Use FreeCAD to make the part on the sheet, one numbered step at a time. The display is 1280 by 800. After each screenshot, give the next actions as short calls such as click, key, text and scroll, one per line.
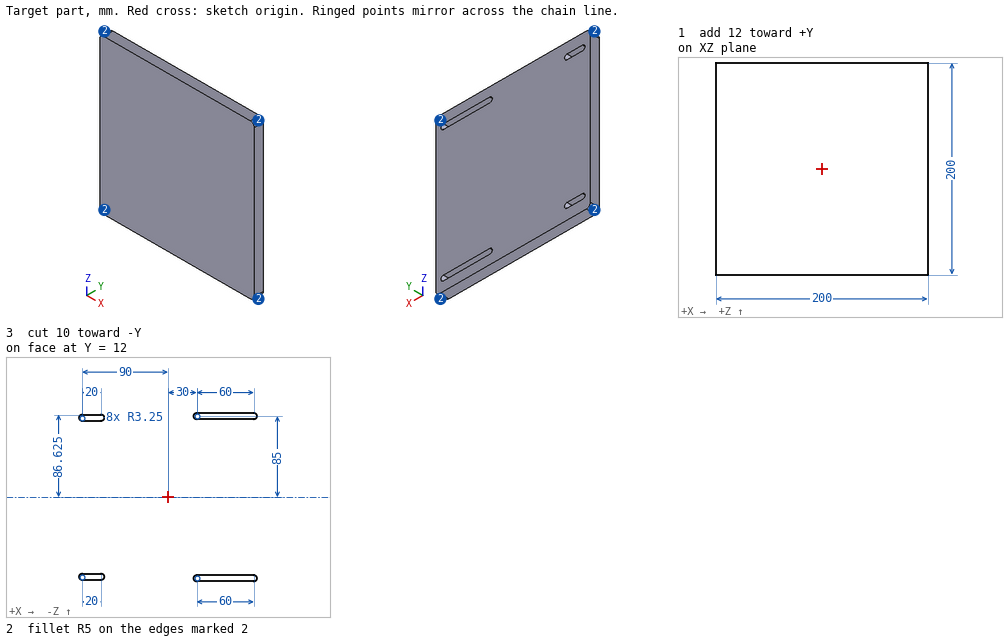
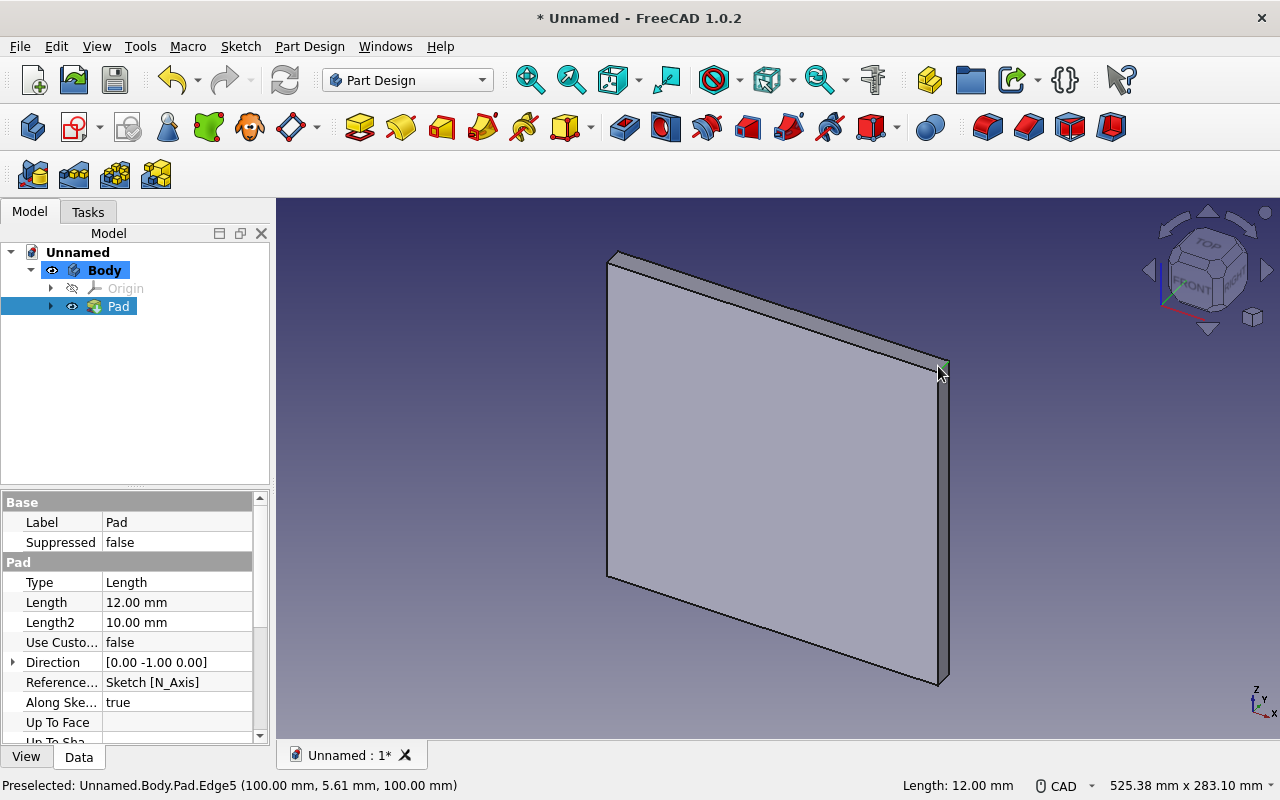
key(0)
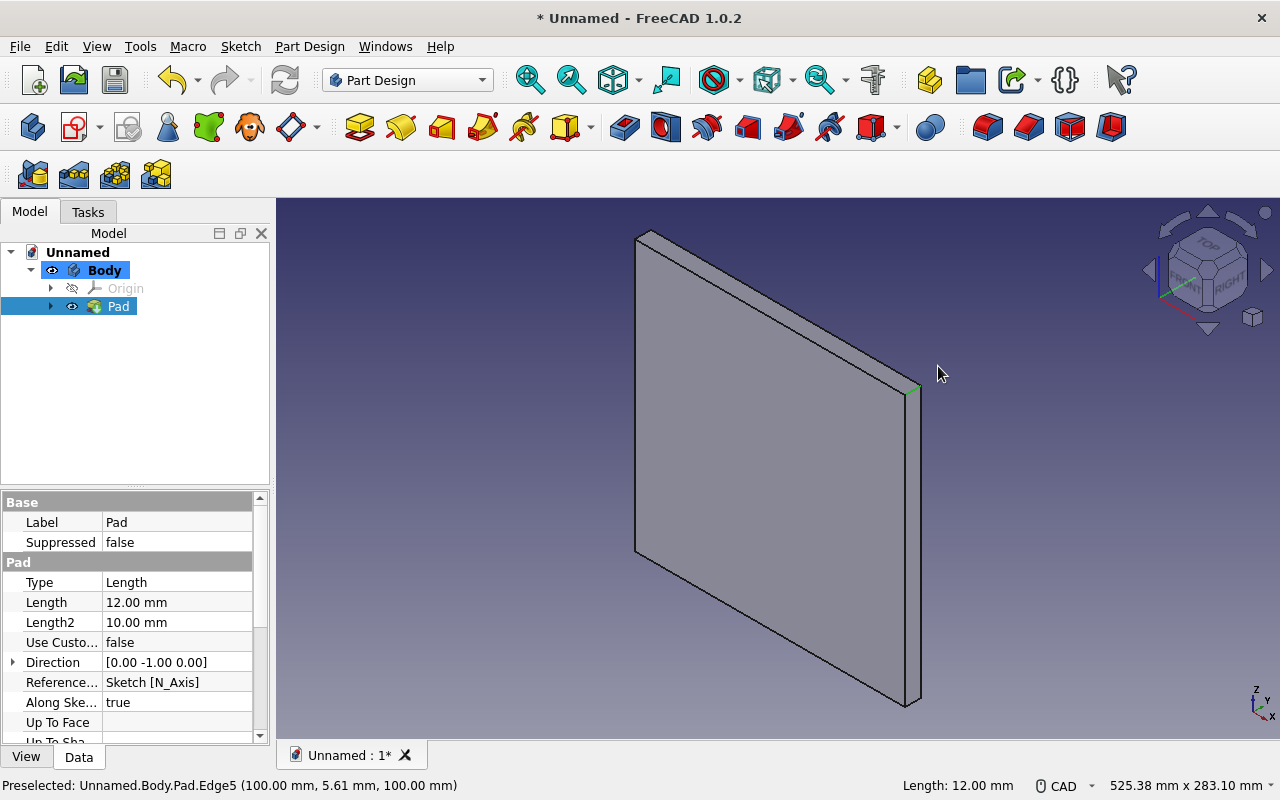
key(2)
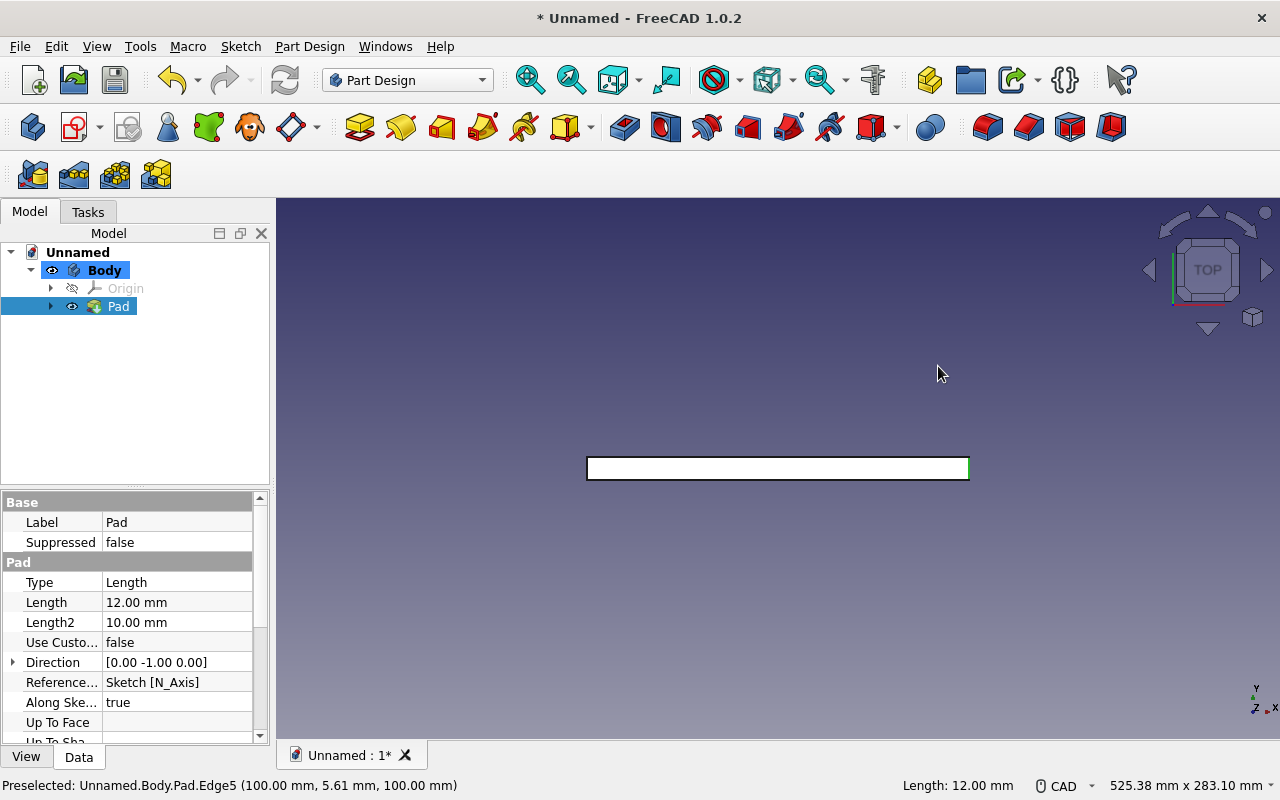
click(531, 80)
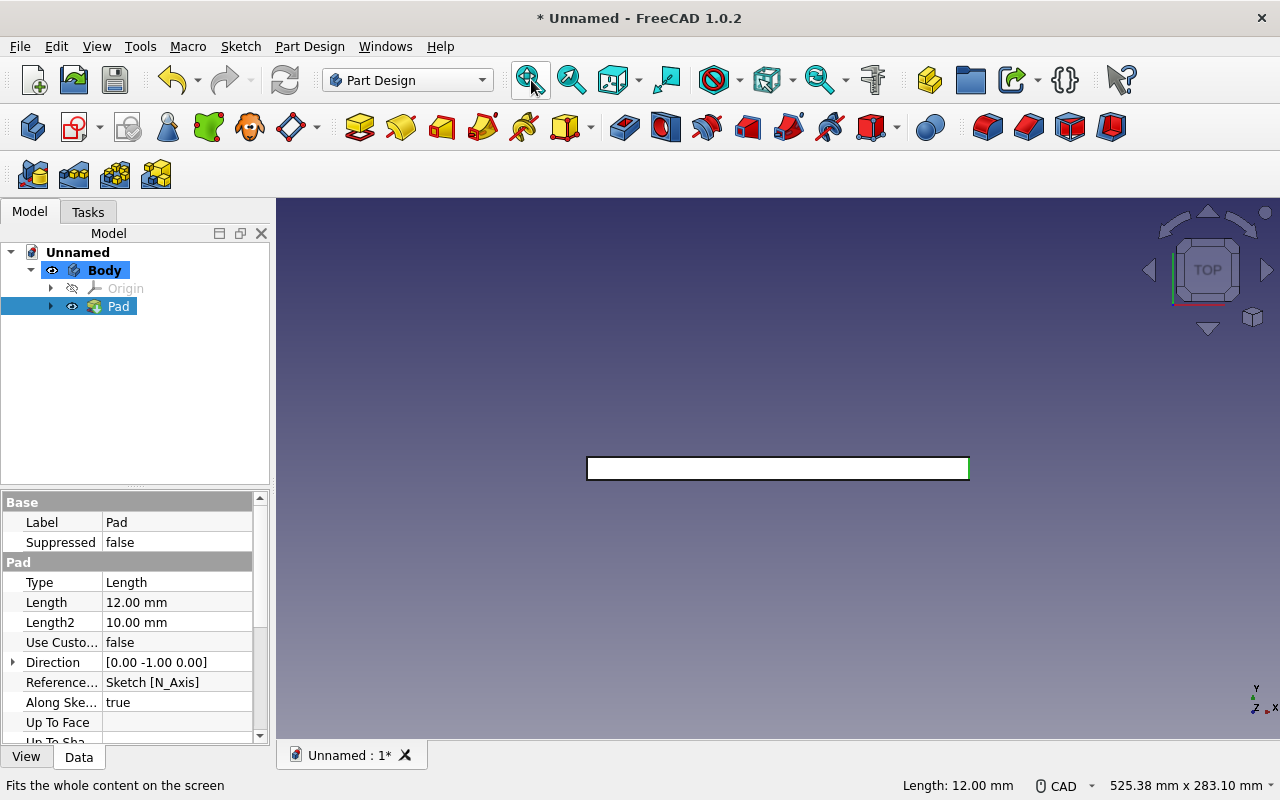
click(587, 467, ctrl)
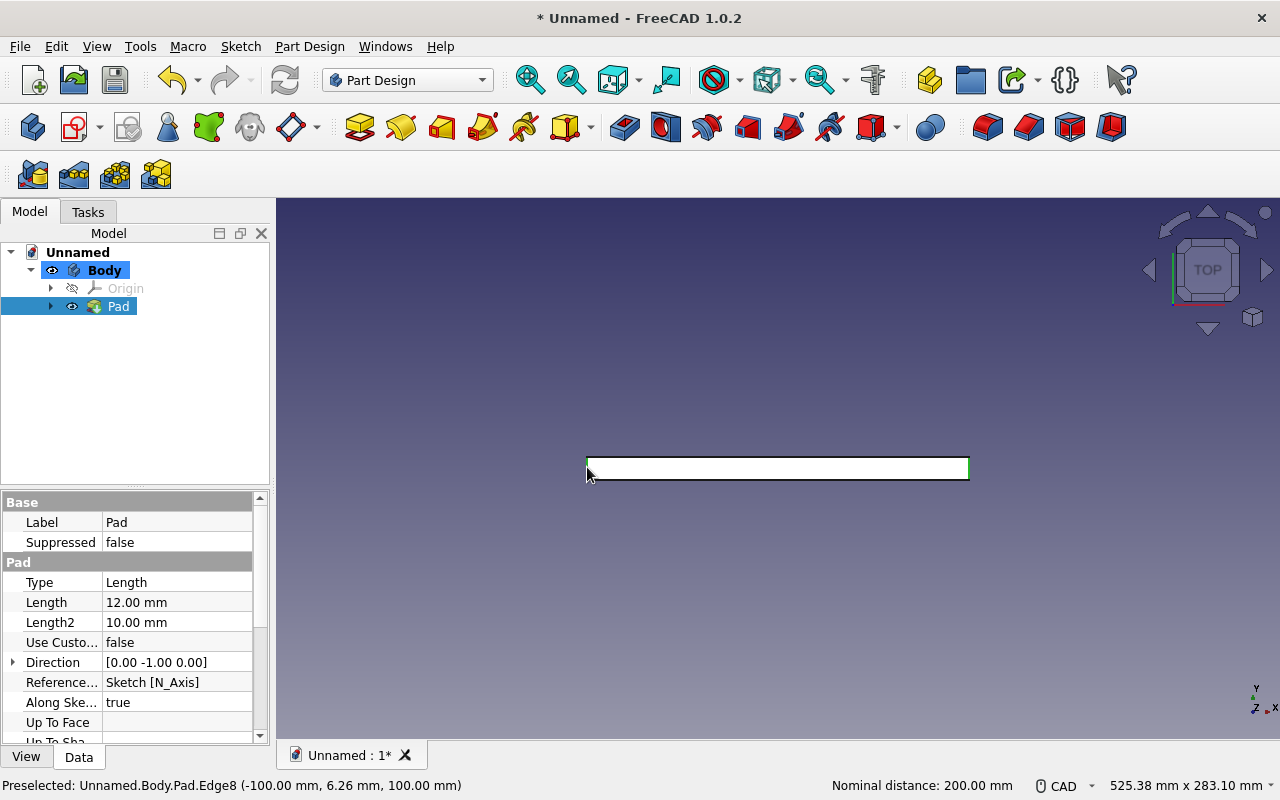
key(1)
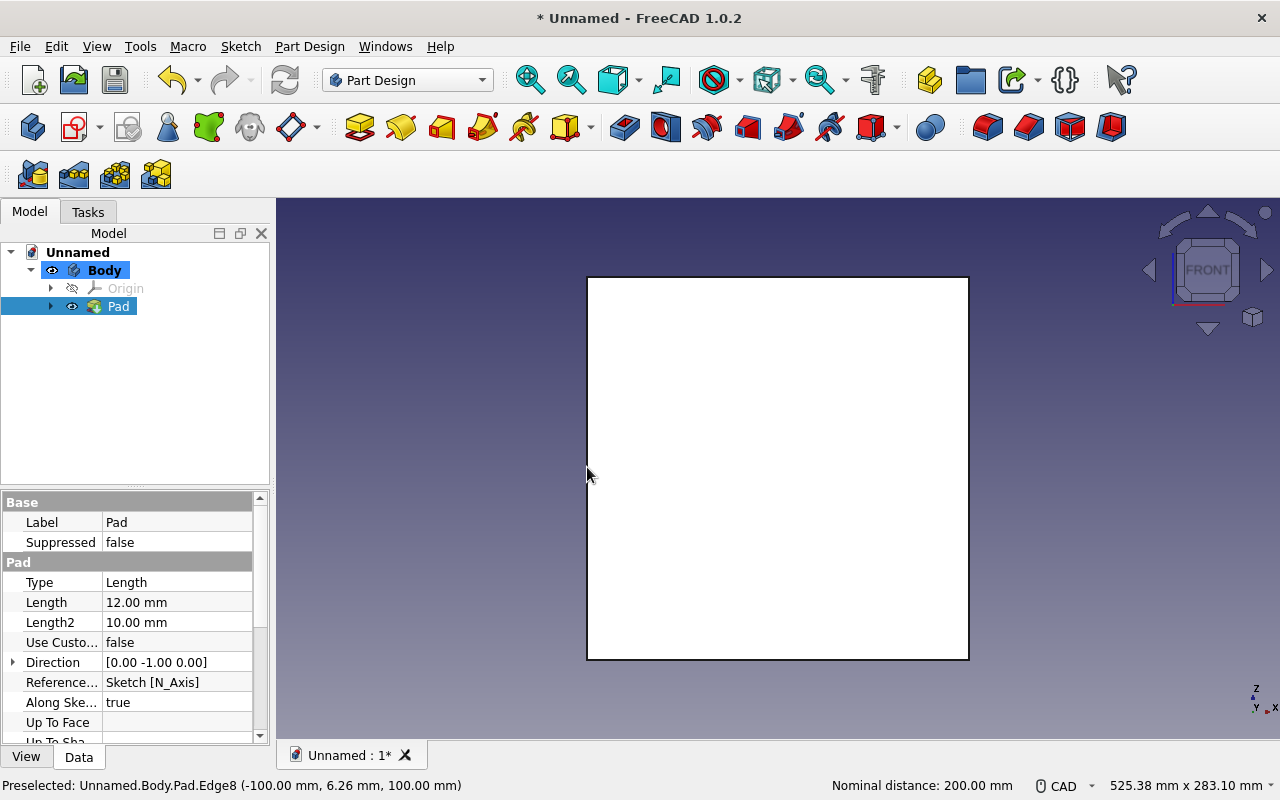
key(3)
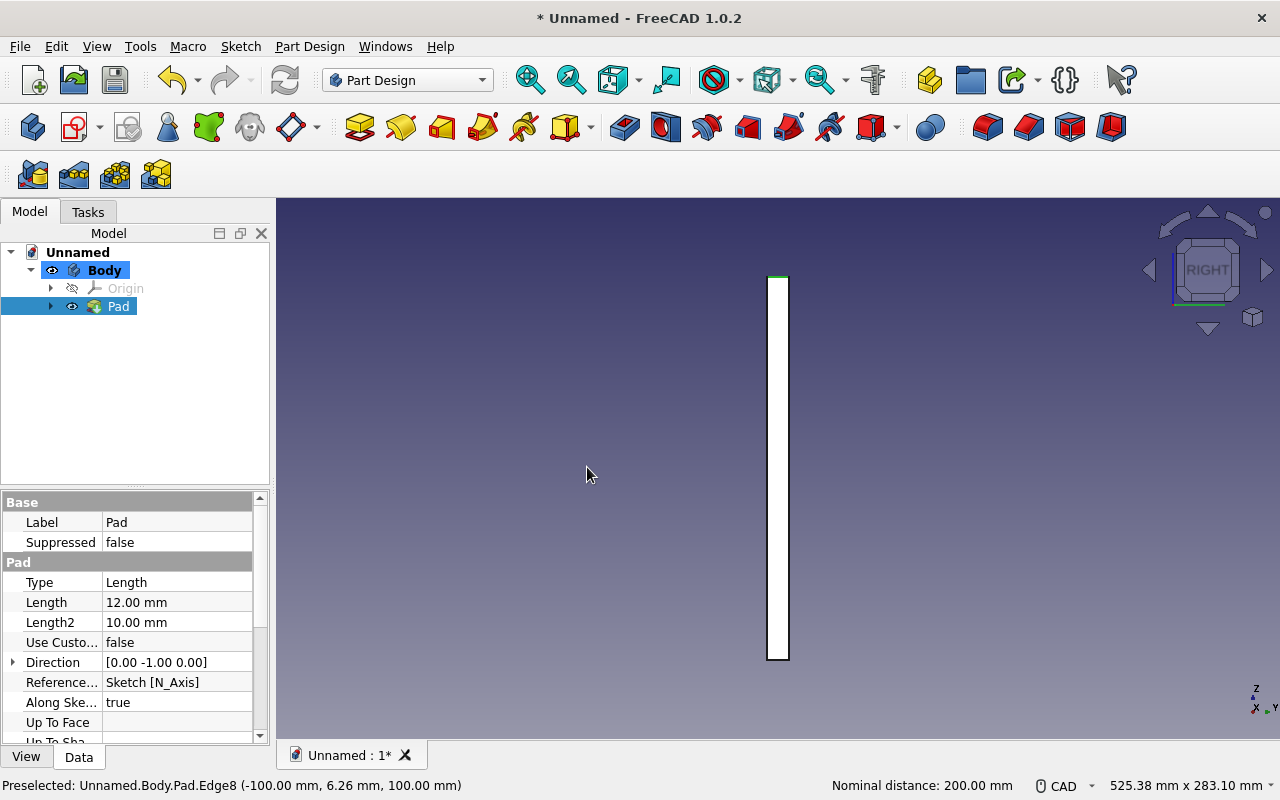
click(778, 659, ctrl)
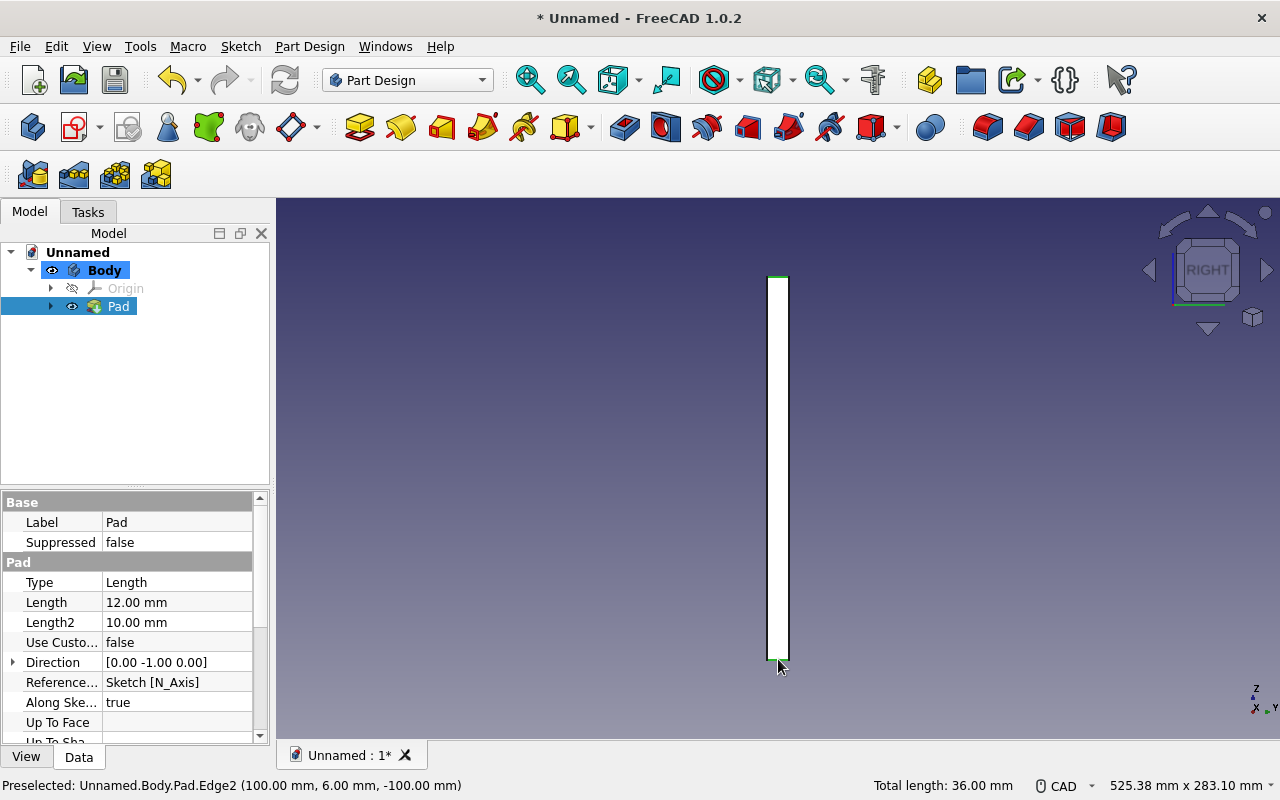
key(5)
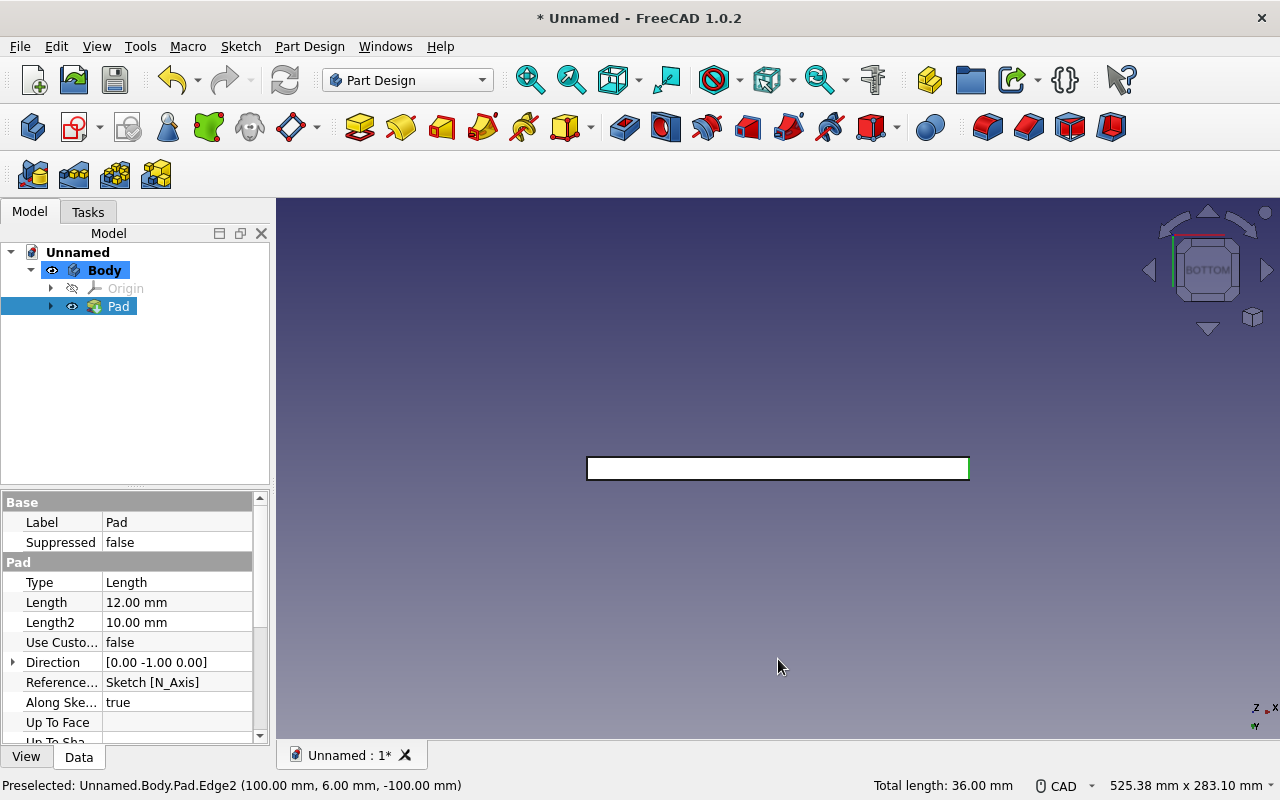
click(531, 80)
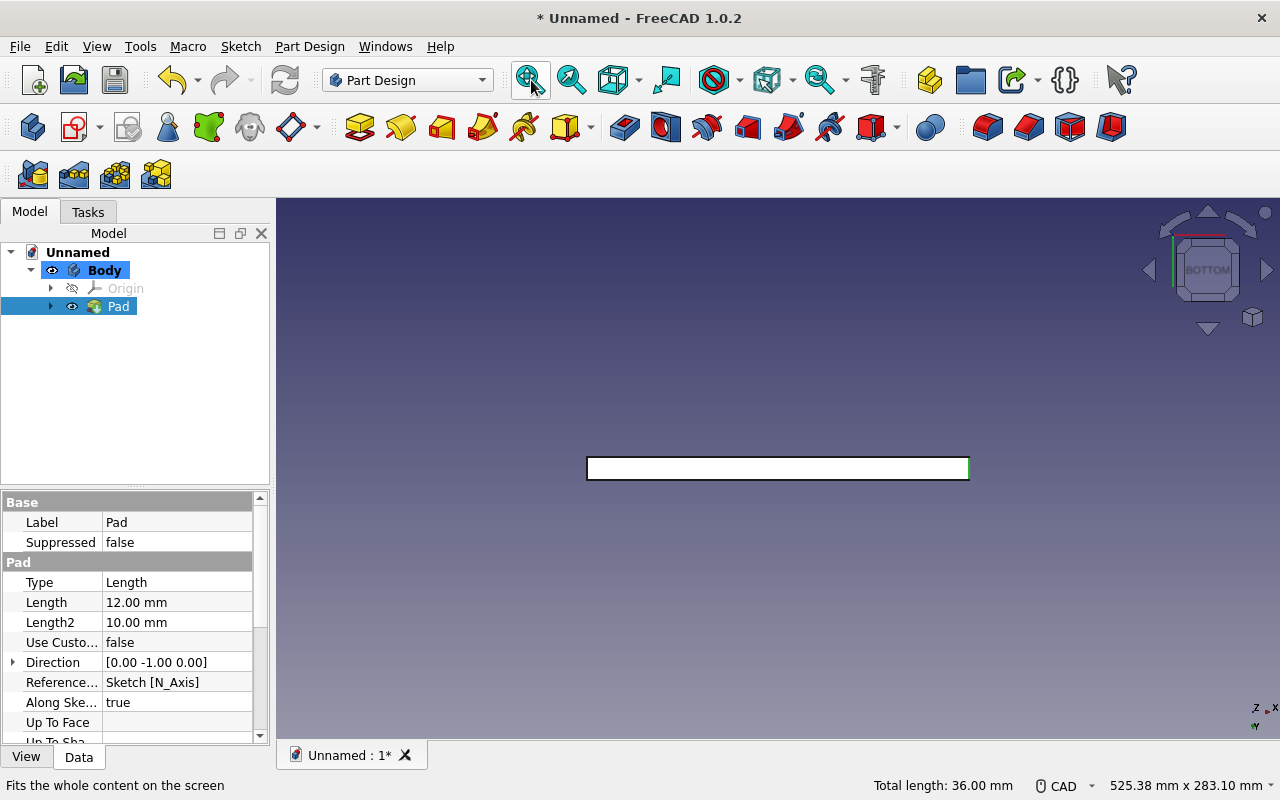
click(587, 467, ctrl)